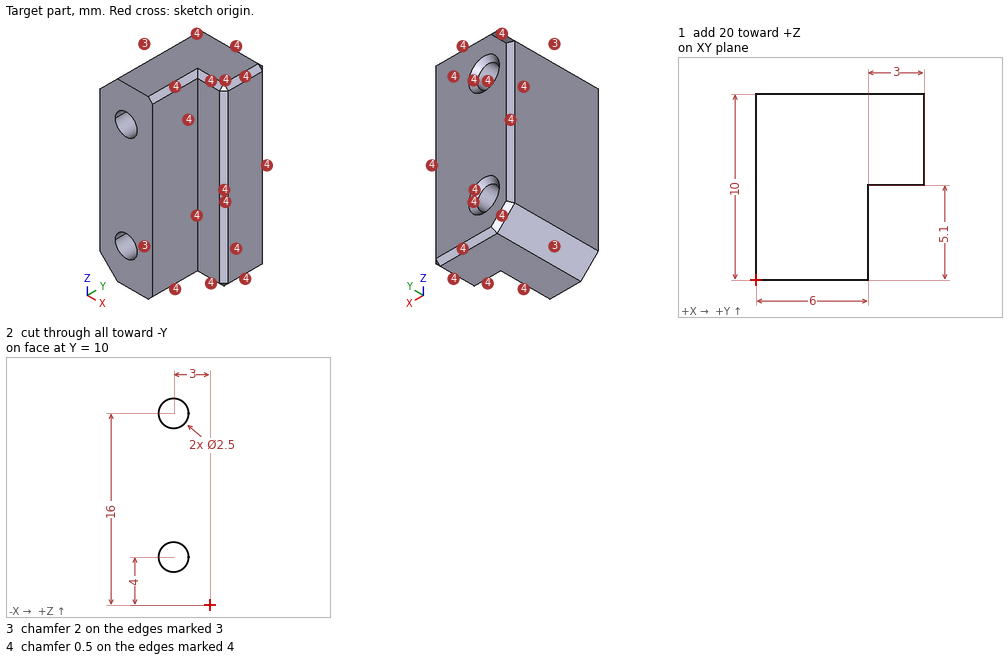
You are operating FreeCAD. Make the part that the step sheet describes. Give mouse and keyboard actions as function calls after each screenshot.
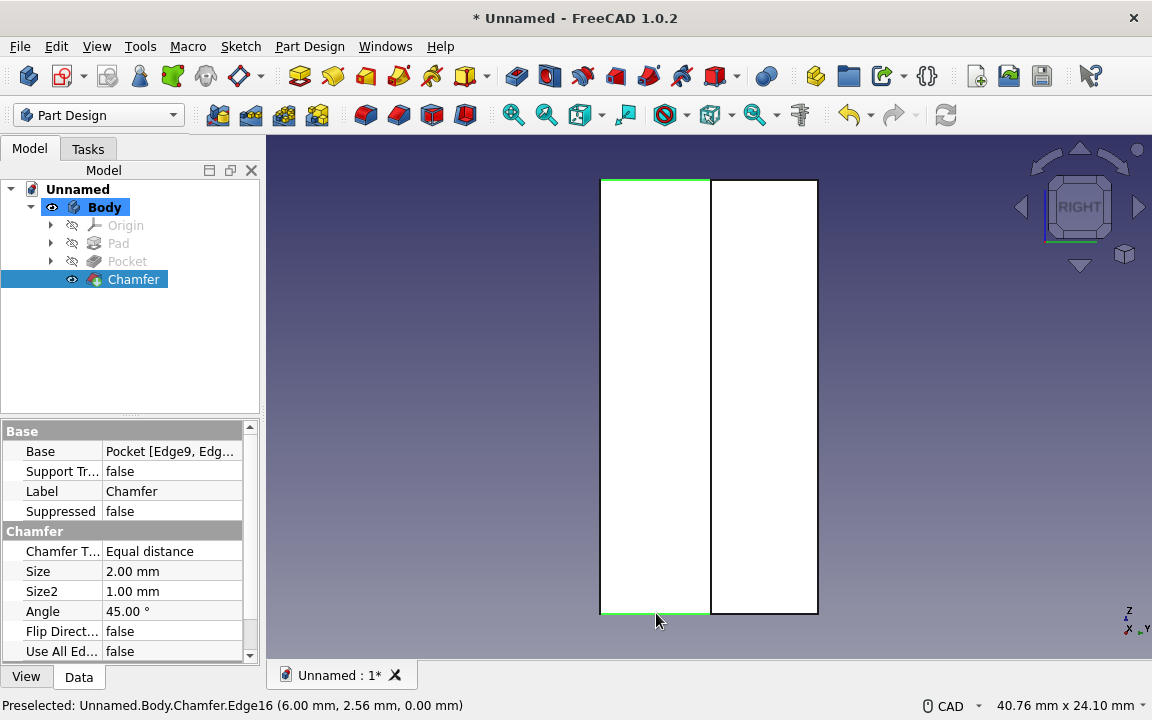
key(5)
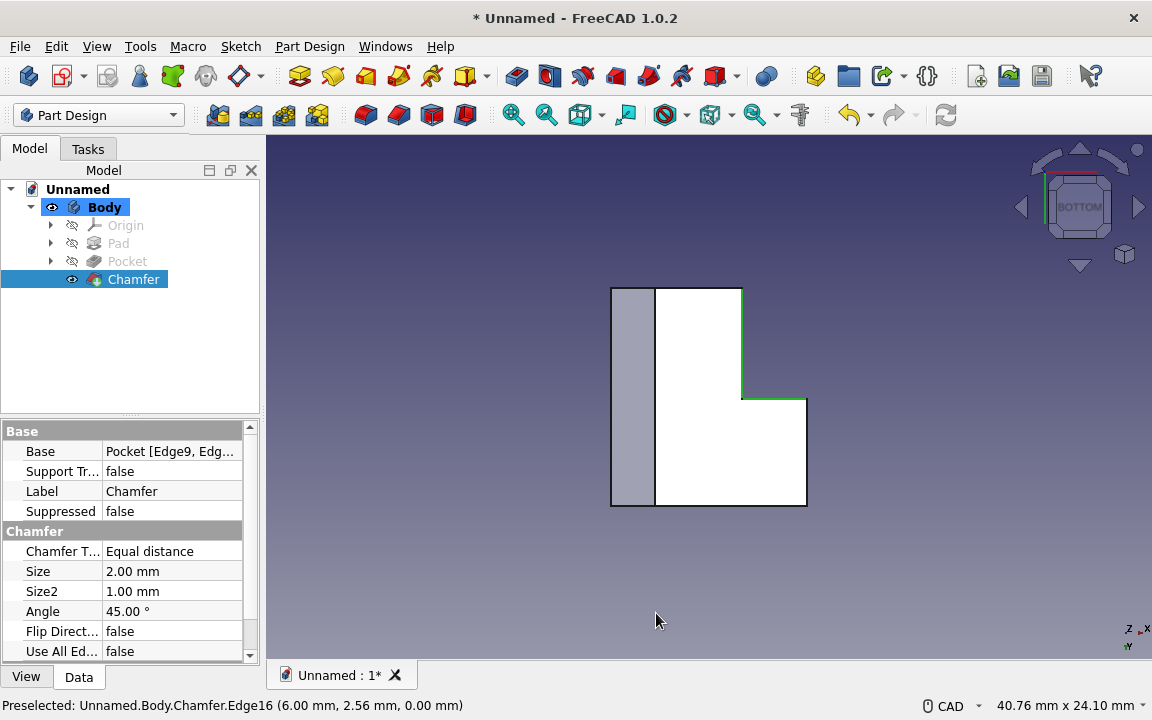
key(v)
key(f)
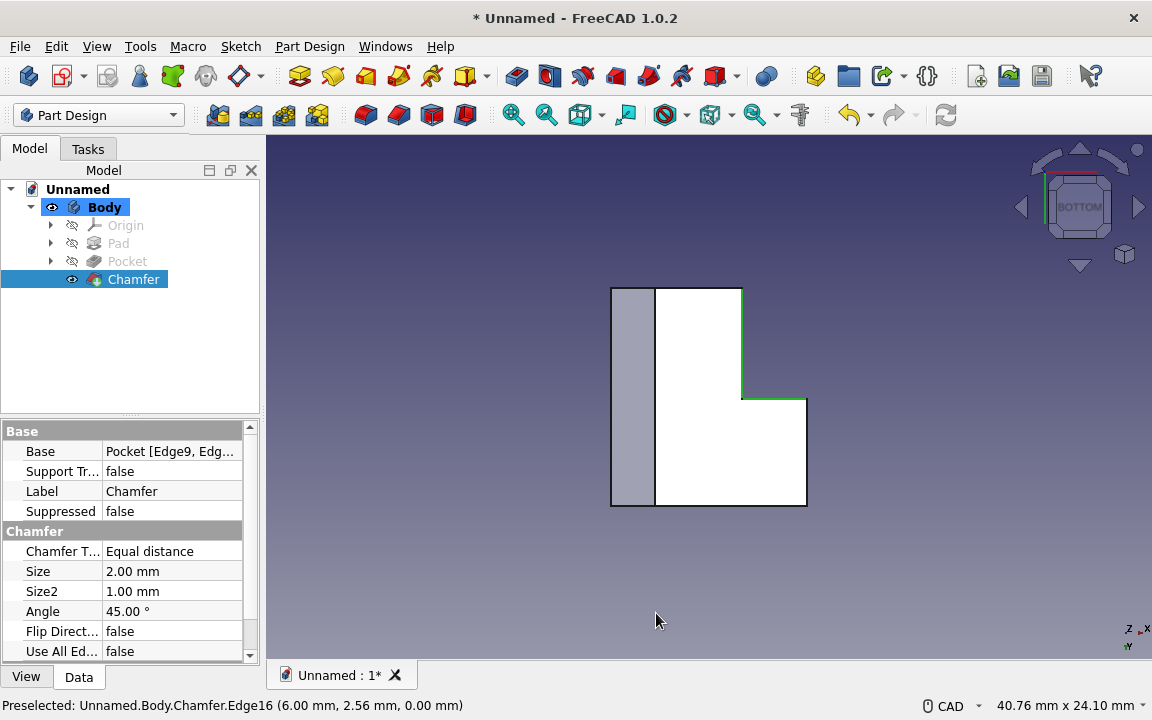
key(4)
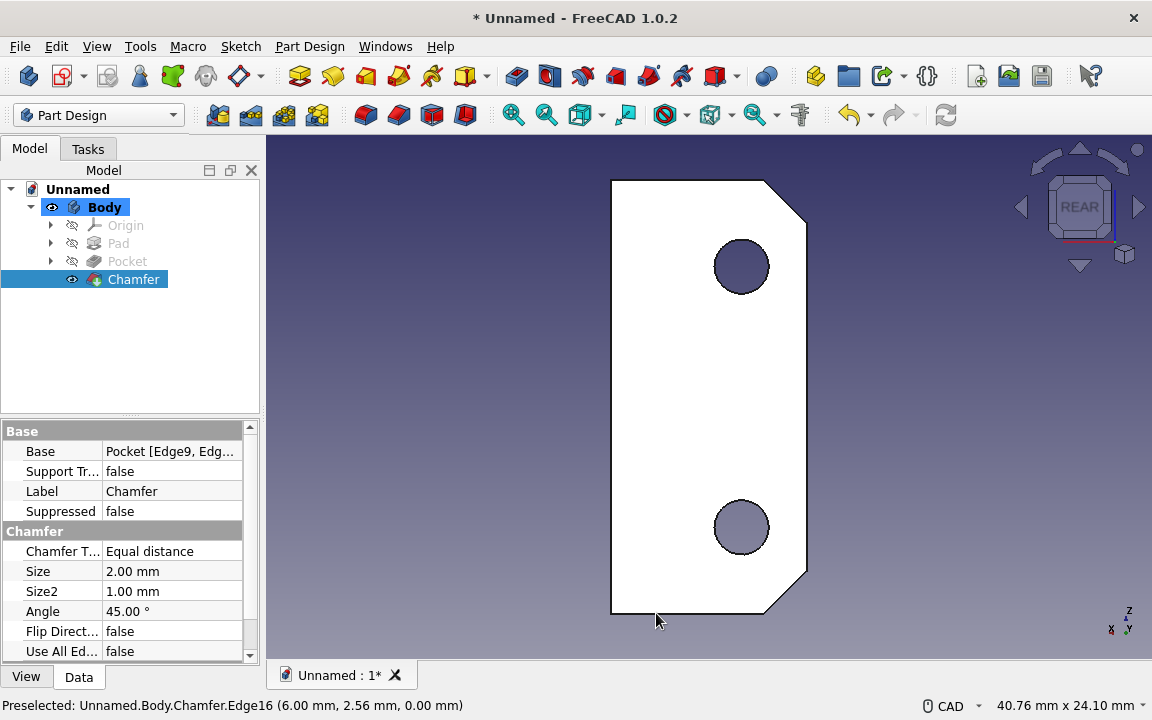
click(709, 396, ctrl)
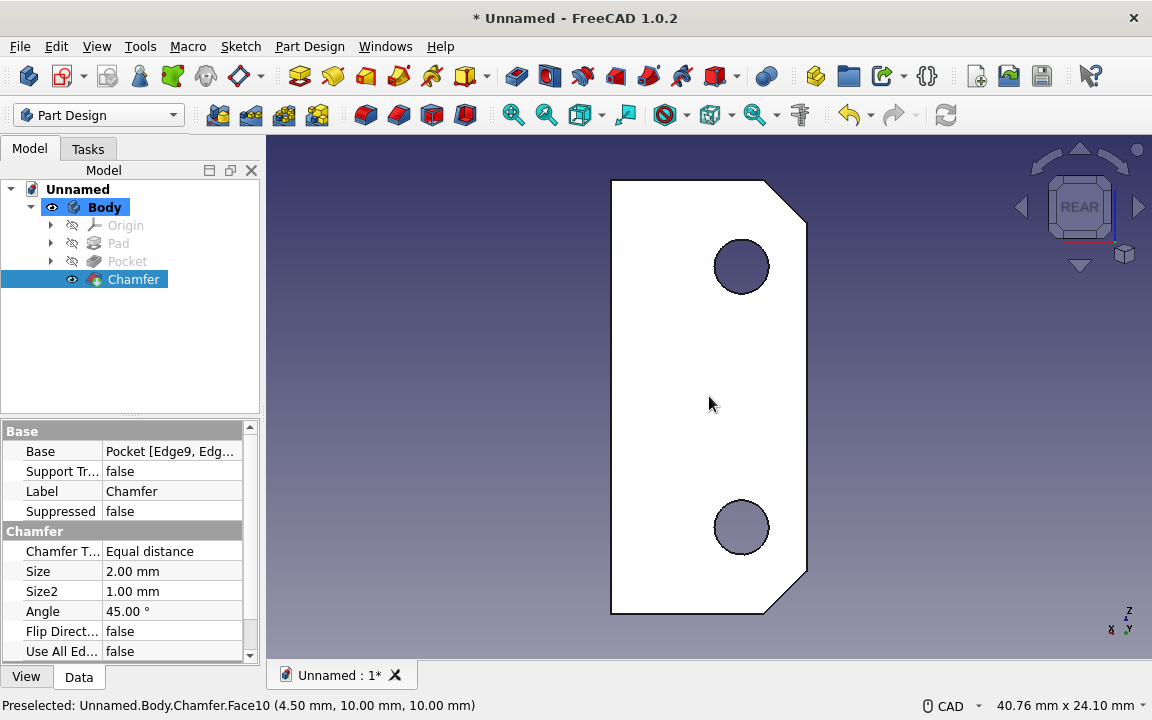
click(399, 116)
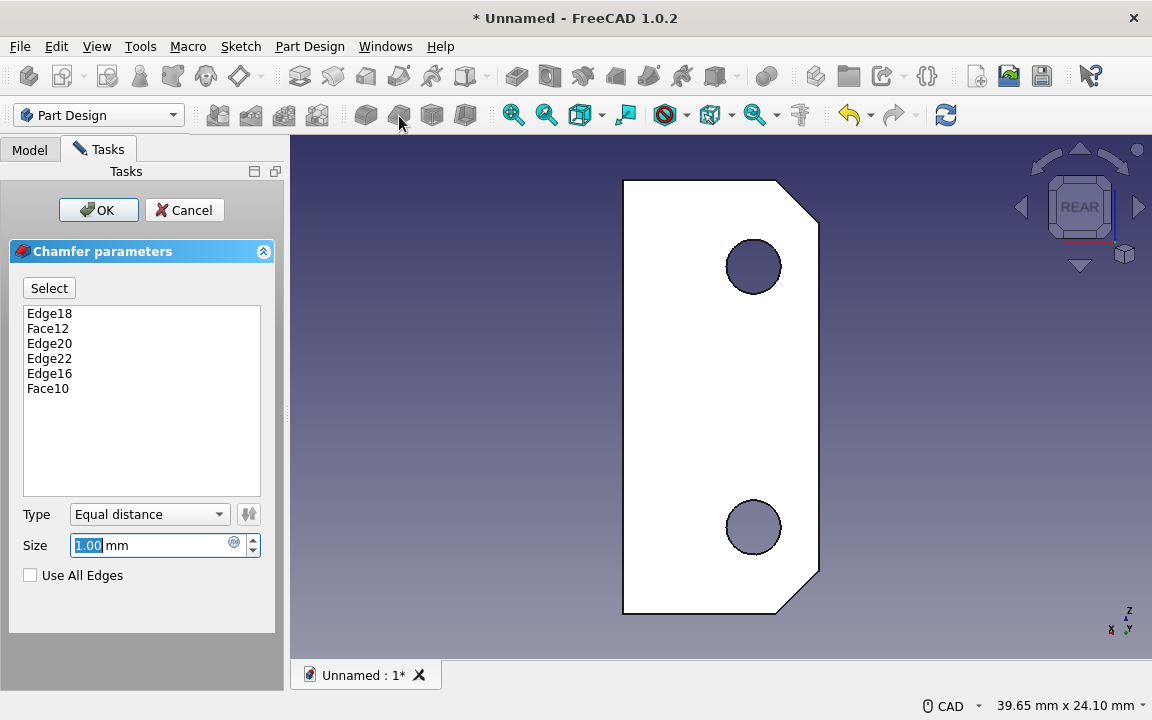
text(0.5)
key(Tab)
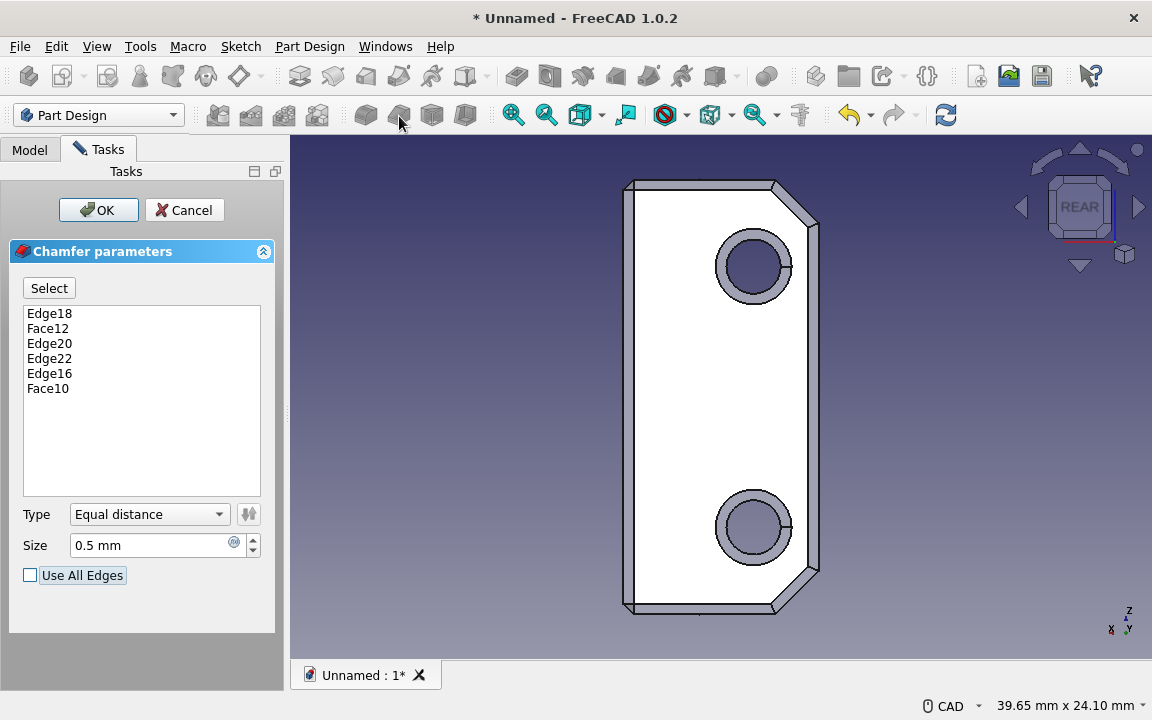
click(99, 210)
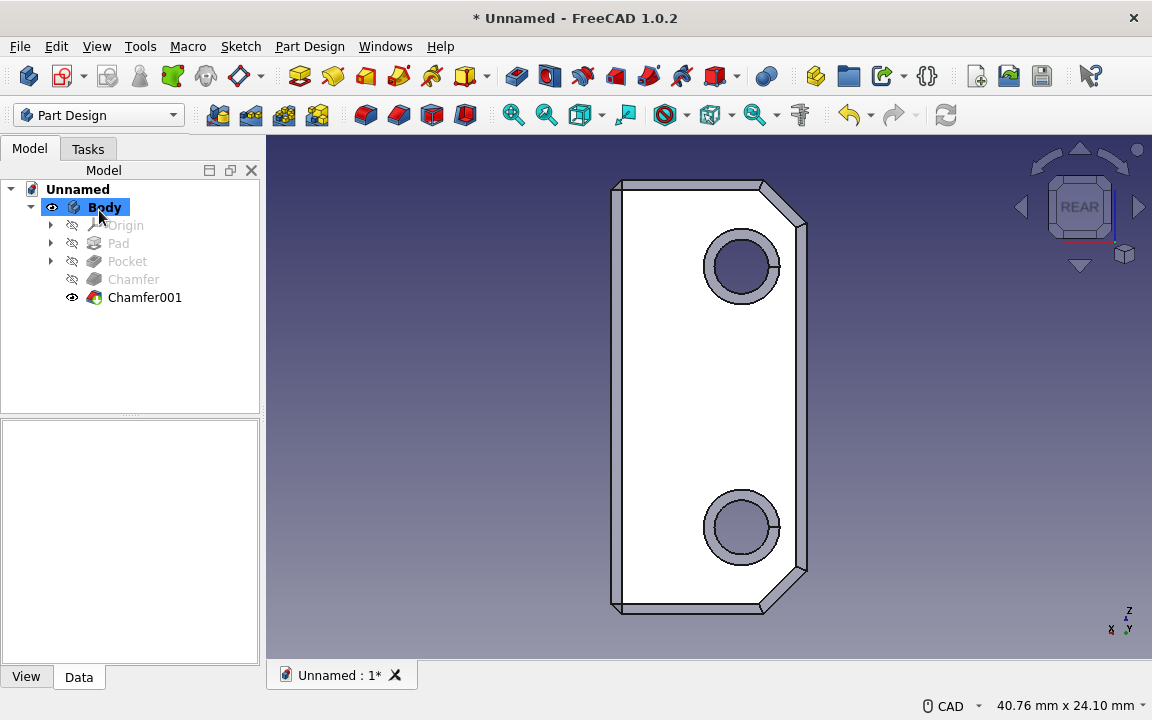
key(0)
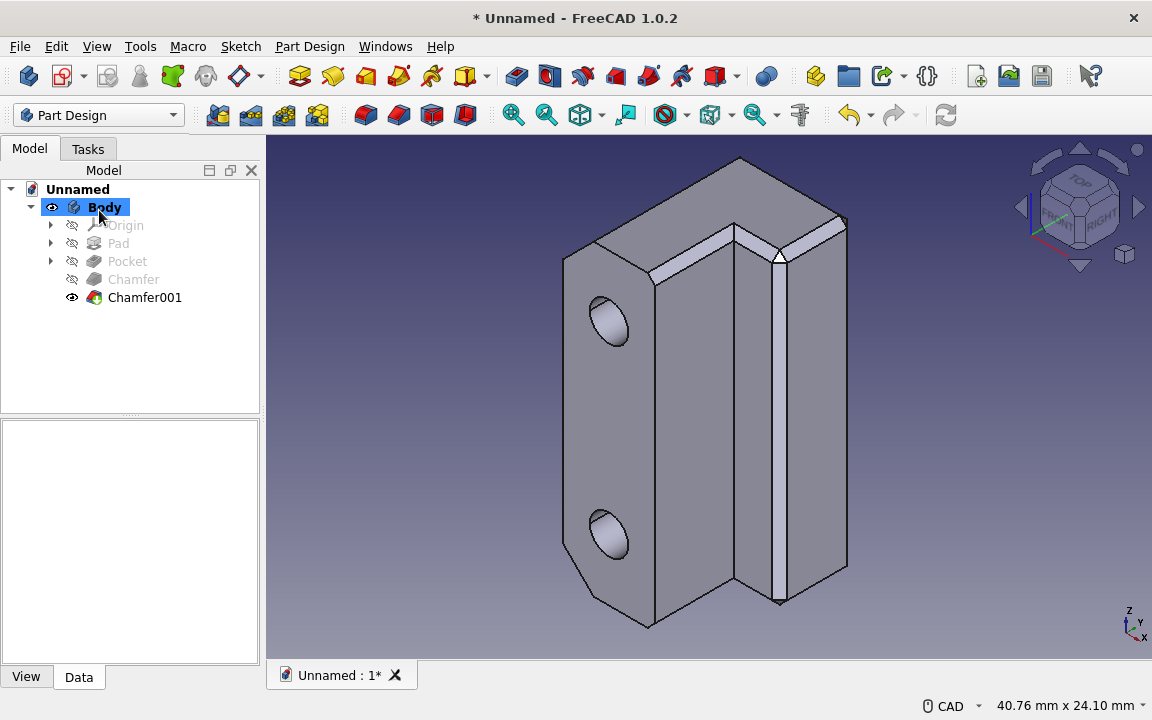
click(514, 116)